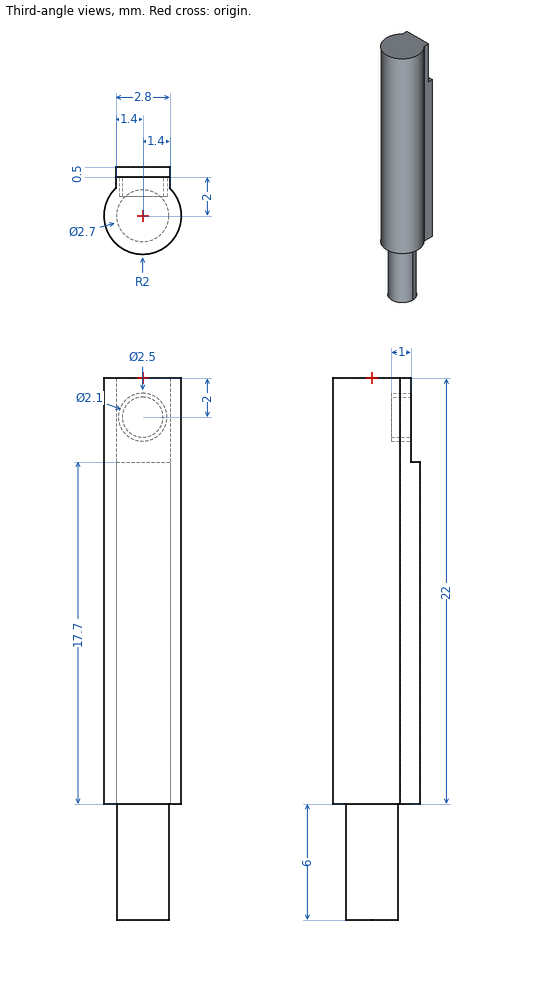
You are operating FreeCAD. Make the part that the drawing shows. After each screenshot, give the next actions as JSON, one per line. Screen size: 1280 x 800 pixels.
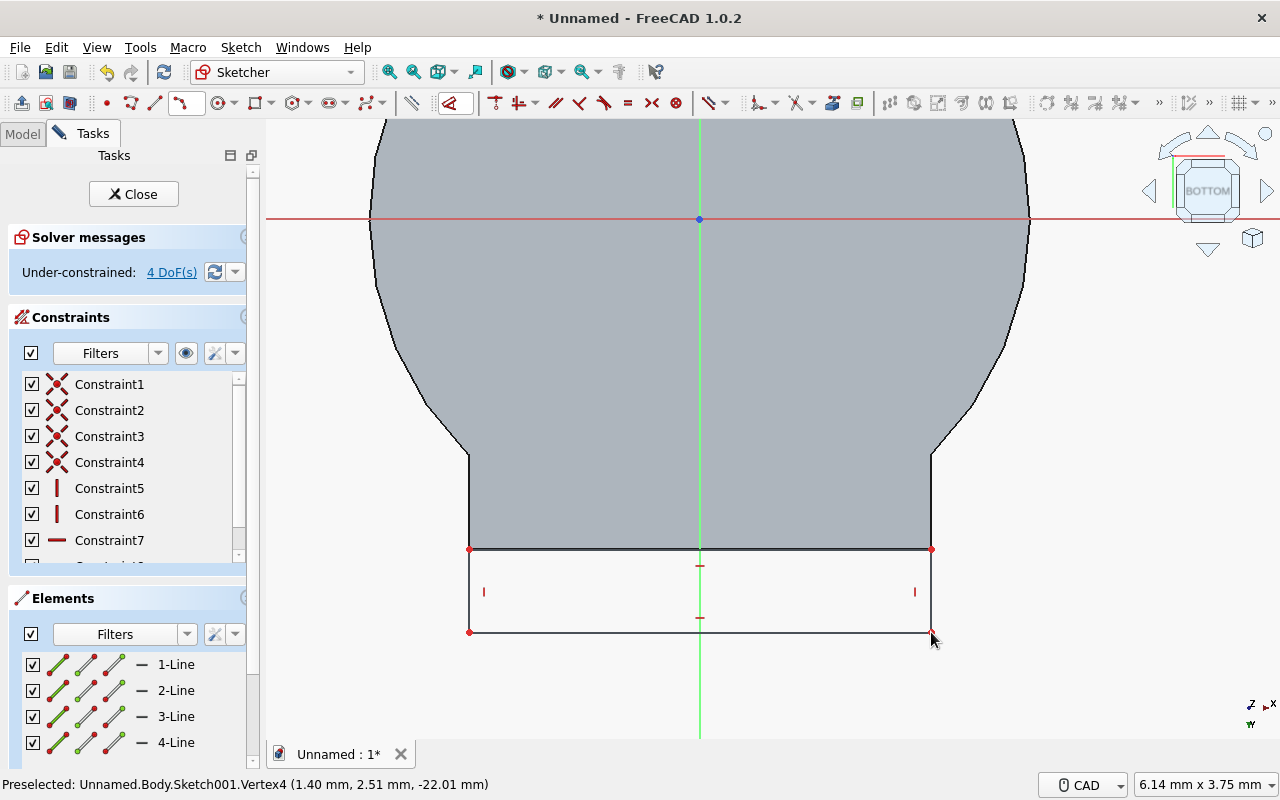
{"action": "left_click", "coordinate": [469, 550]}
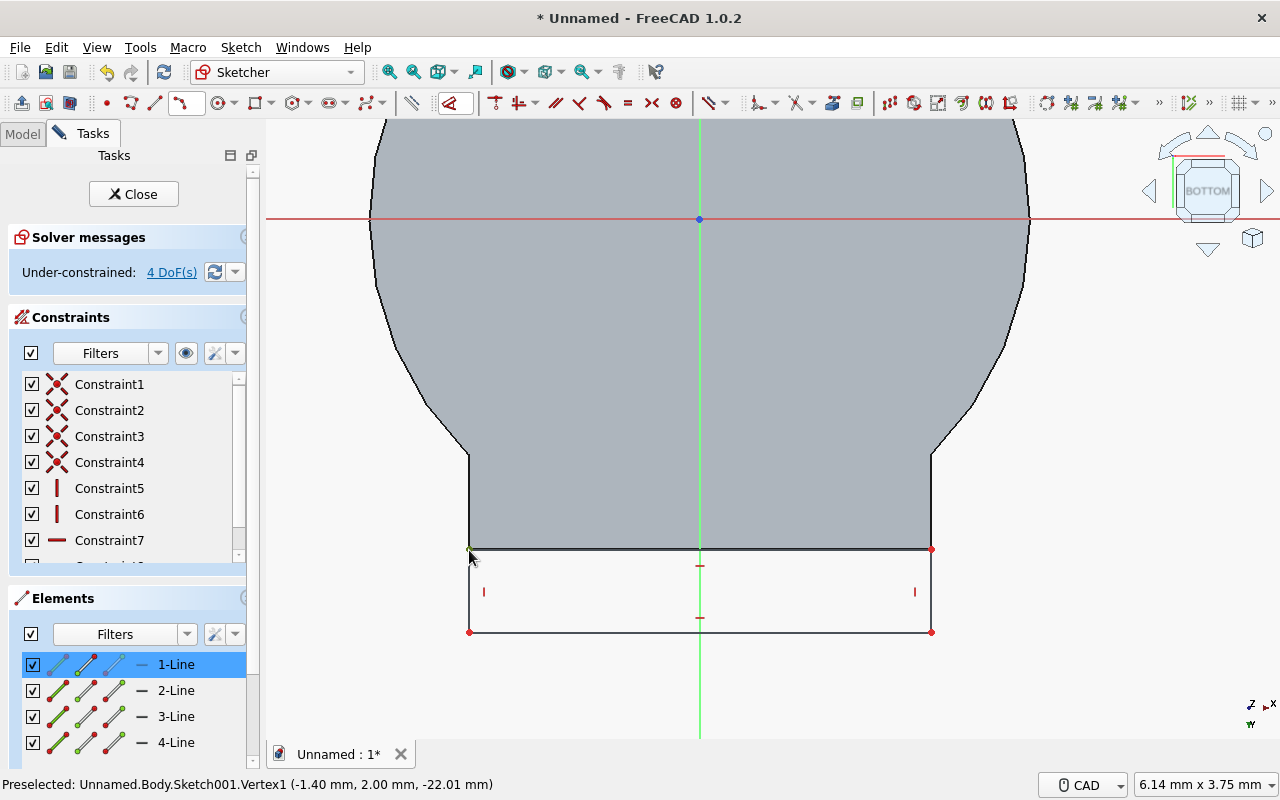
{"action": "left_click", "coordinate": [468, 104]}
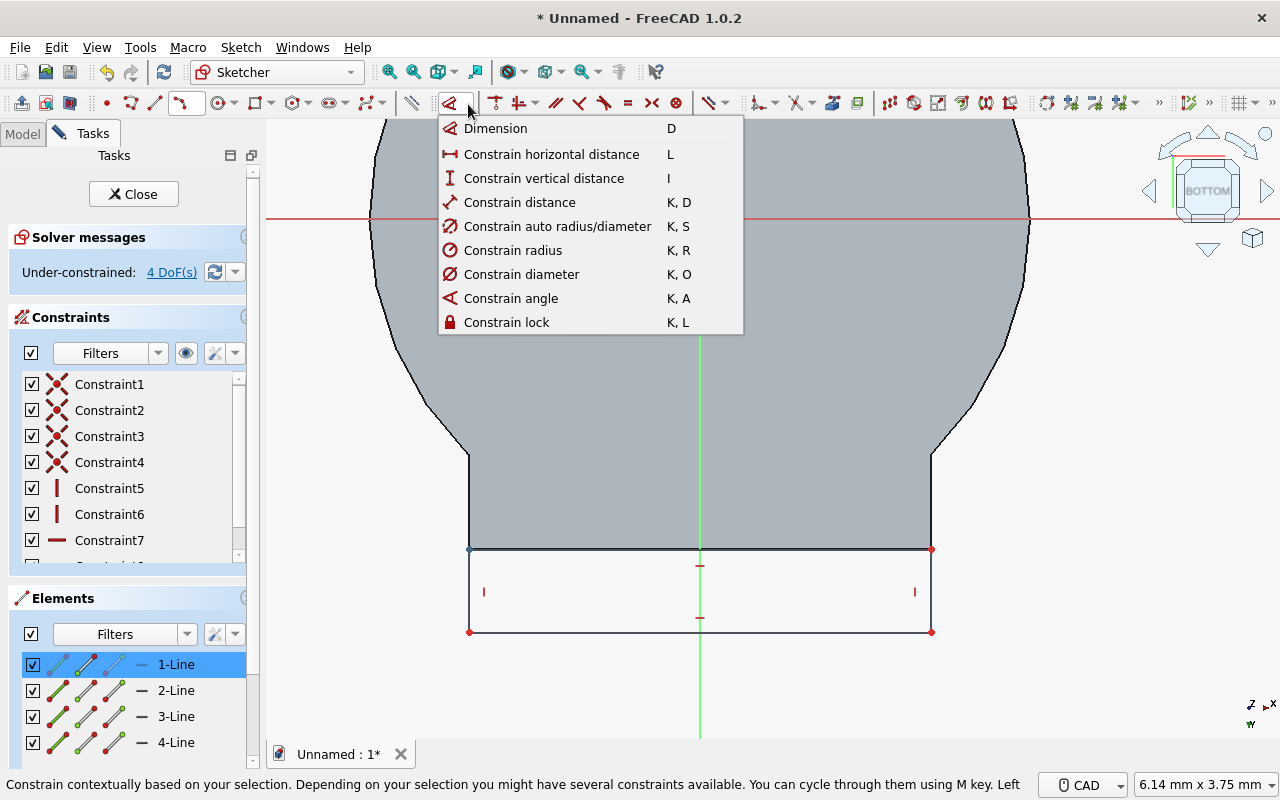
{"action": "left_click", "coordinate": [591, 178]}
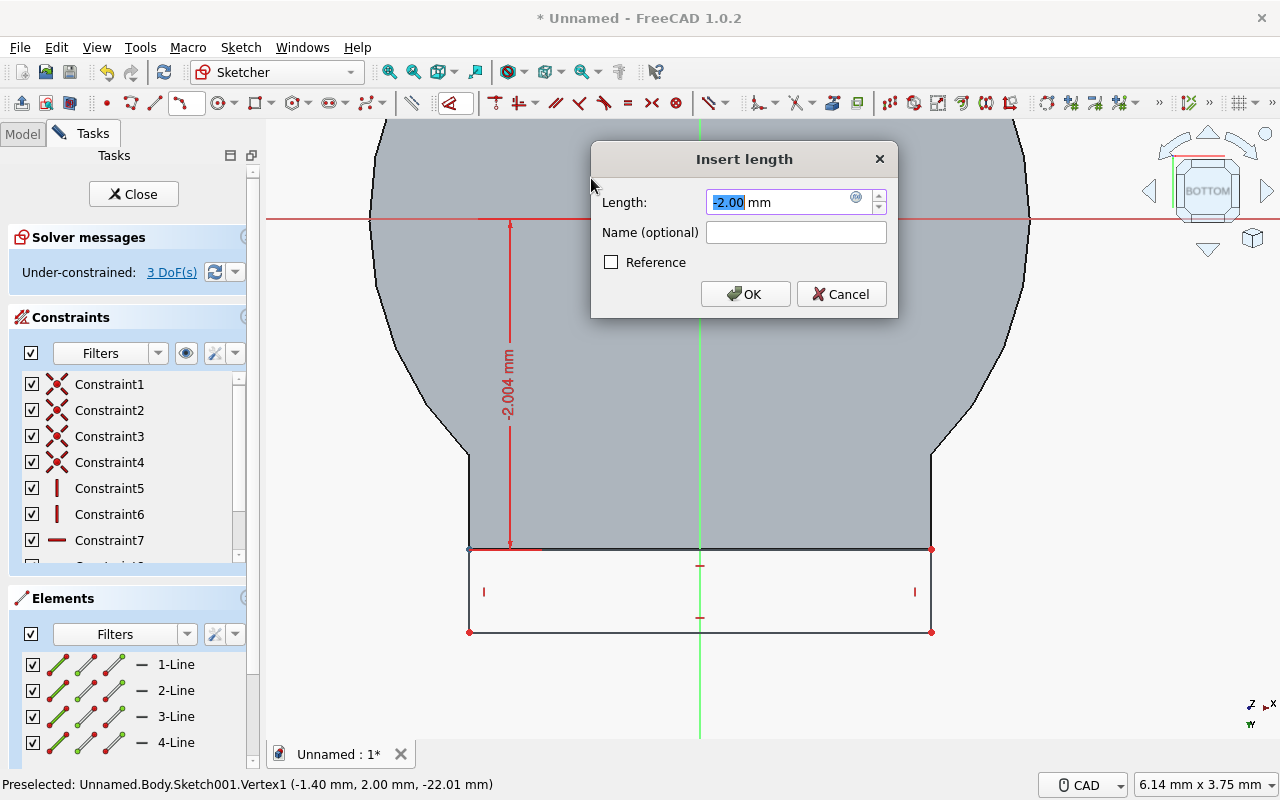
{"action": "type", "text": "-2"}
{"action": "key", "text": "Return"}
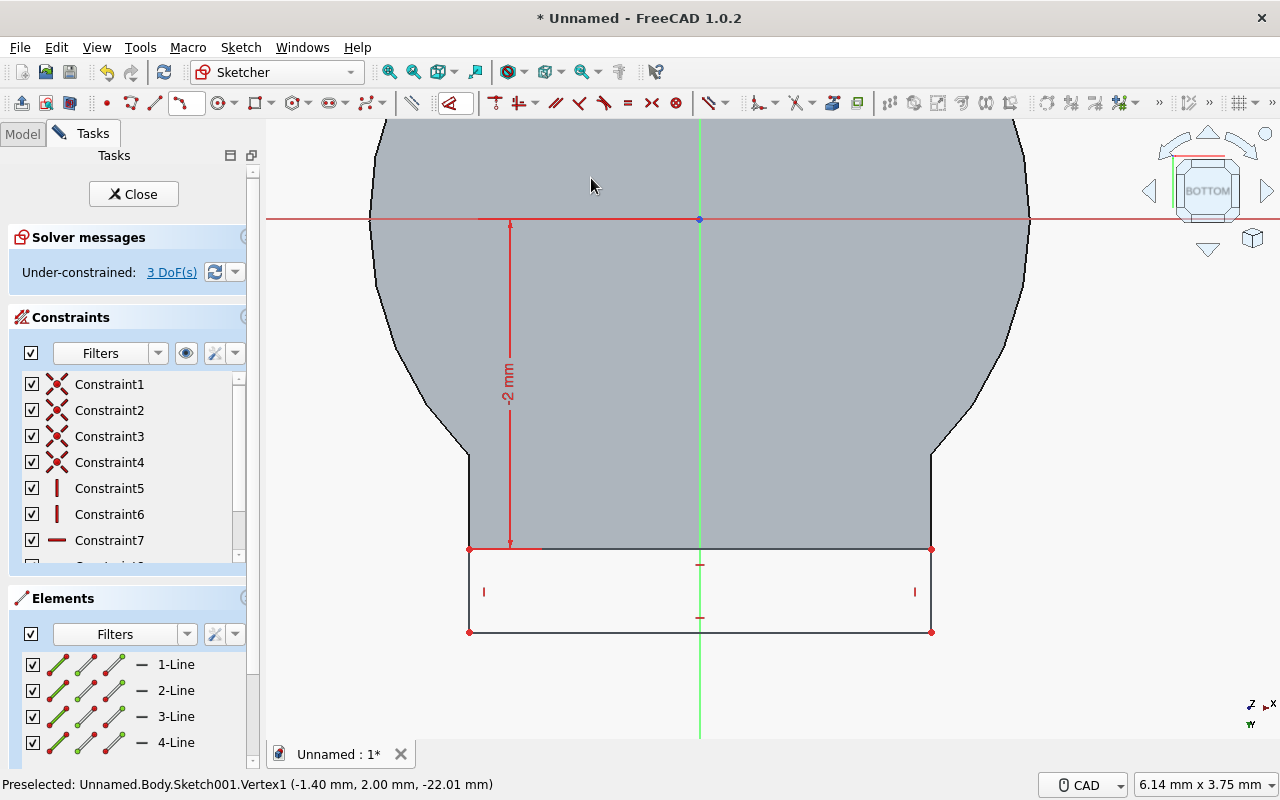
{"action": "left_click", "coordinate": [469, 574]}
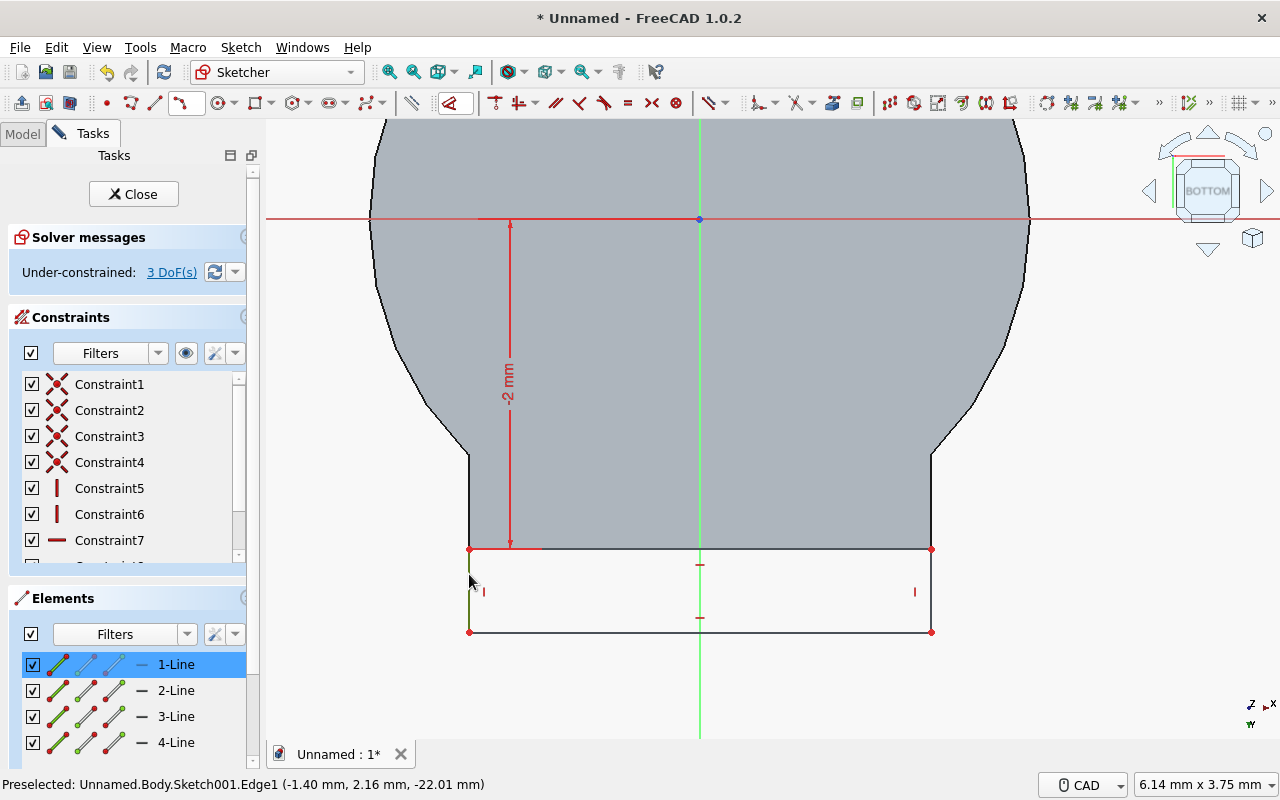
{"action": "key", "text": "i"}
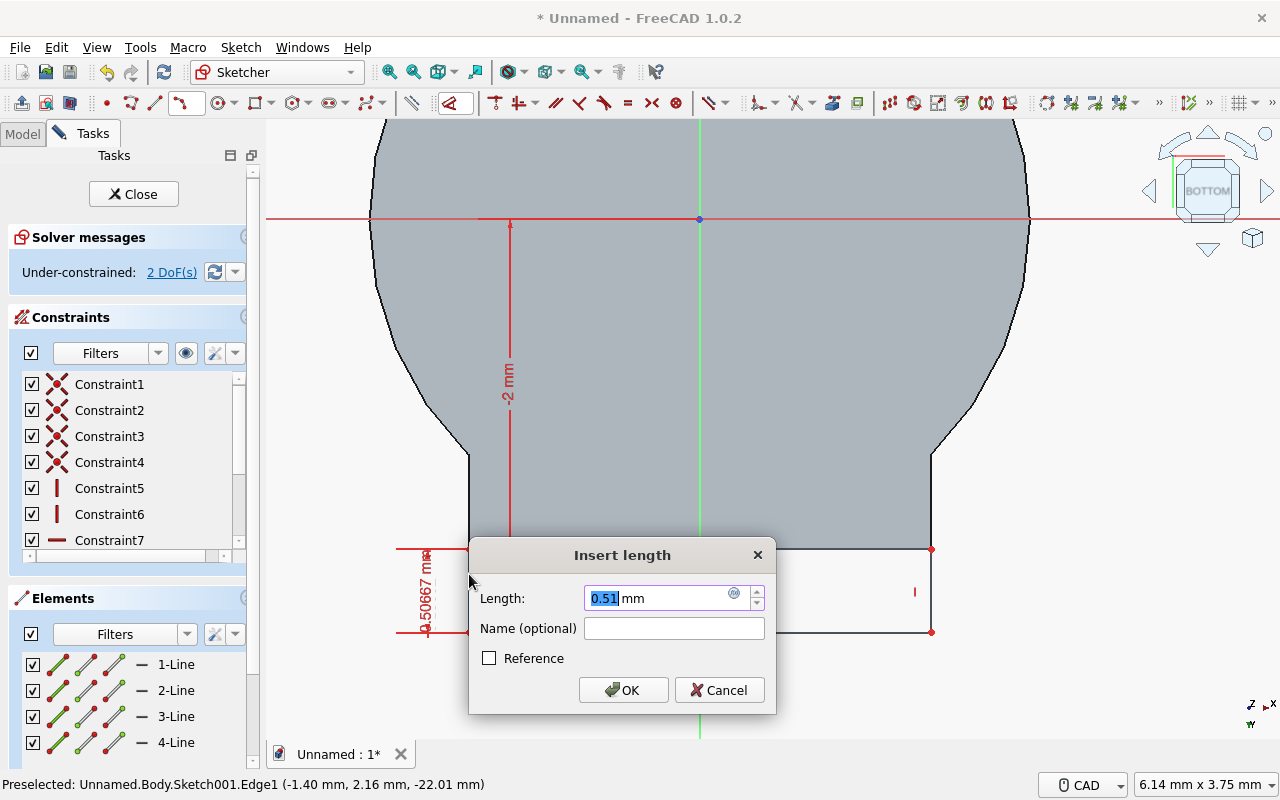
{"action": "type", "text": "0.5"}
{"action": "key", "text": "Return"}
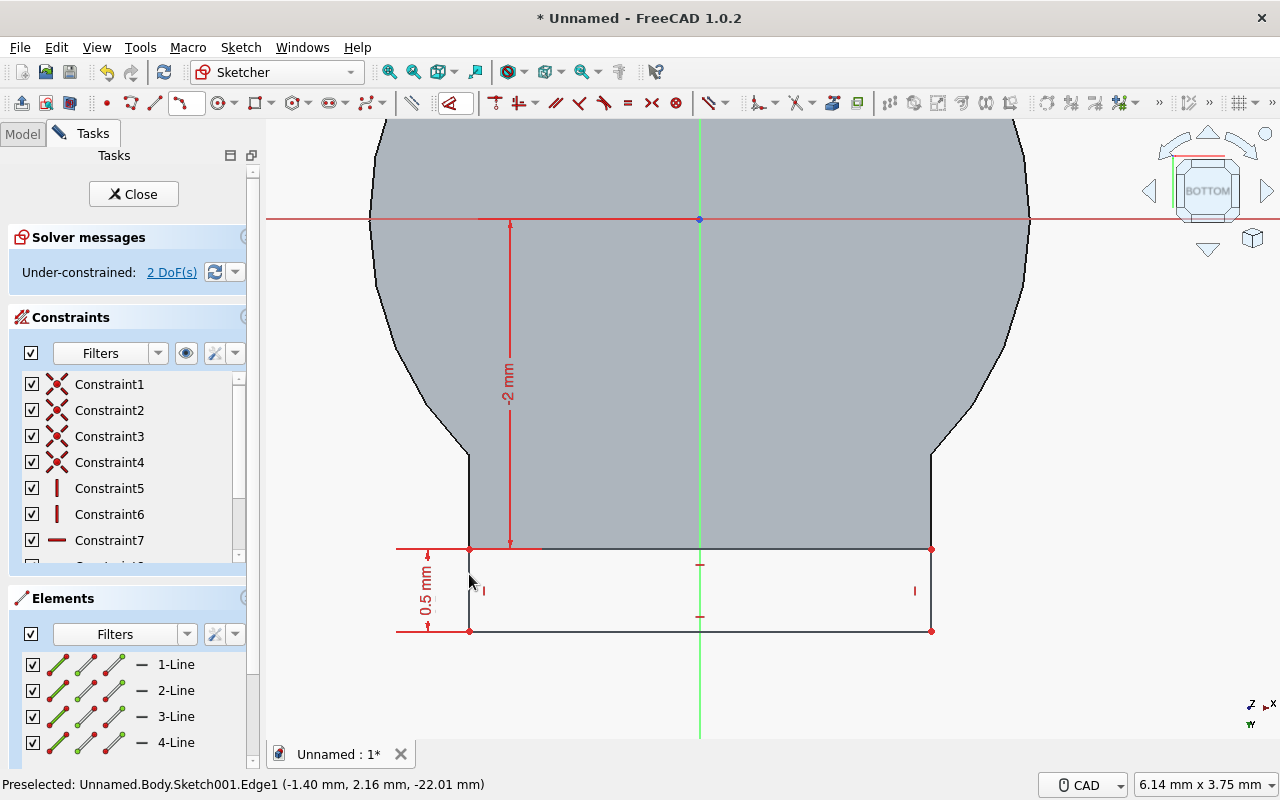
{"action": "left_click", "coordinate": [608, 632]}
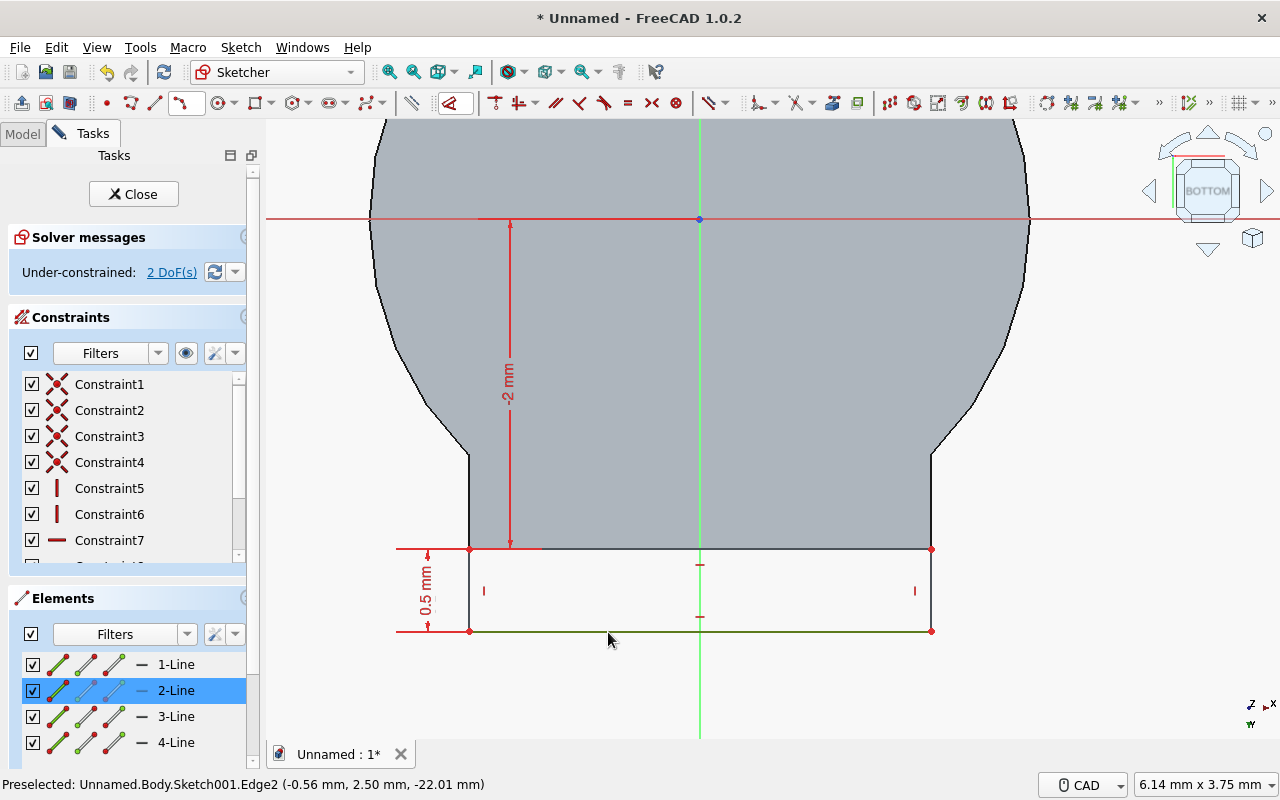
{"action": "left_click", "coordinate": [468, 104]}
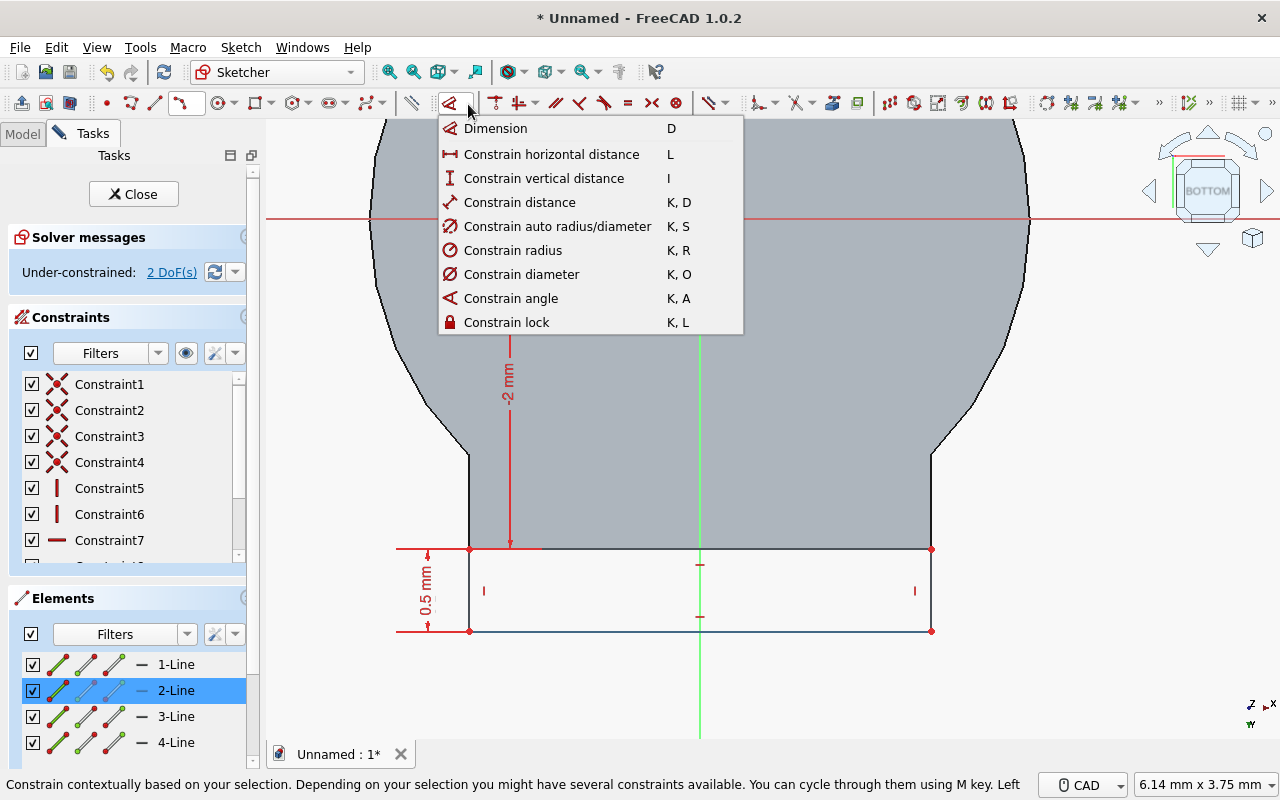
{"action": "left_click", "coordinate": [591, 154]}